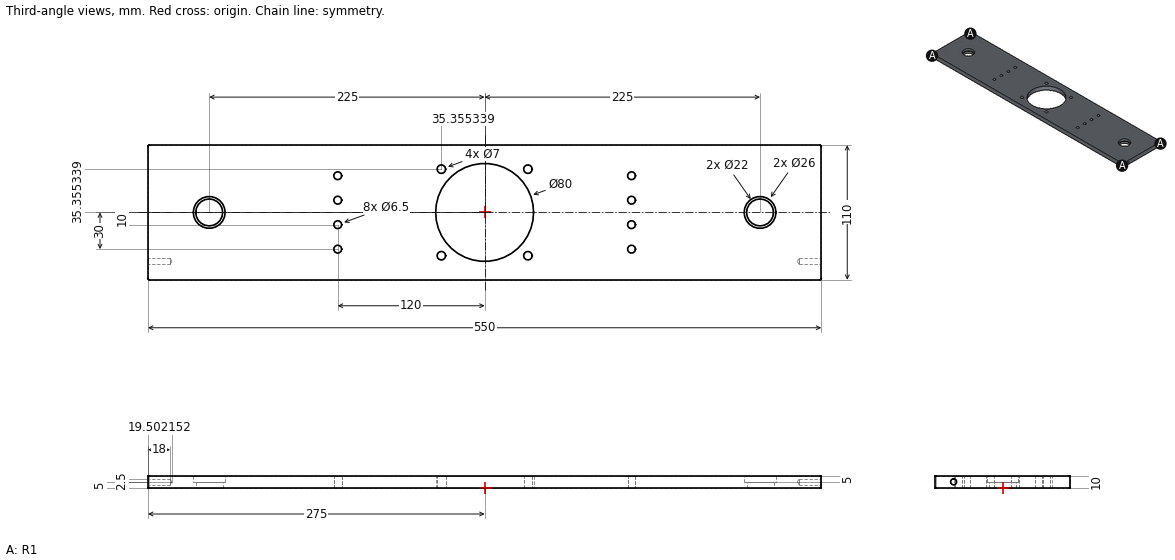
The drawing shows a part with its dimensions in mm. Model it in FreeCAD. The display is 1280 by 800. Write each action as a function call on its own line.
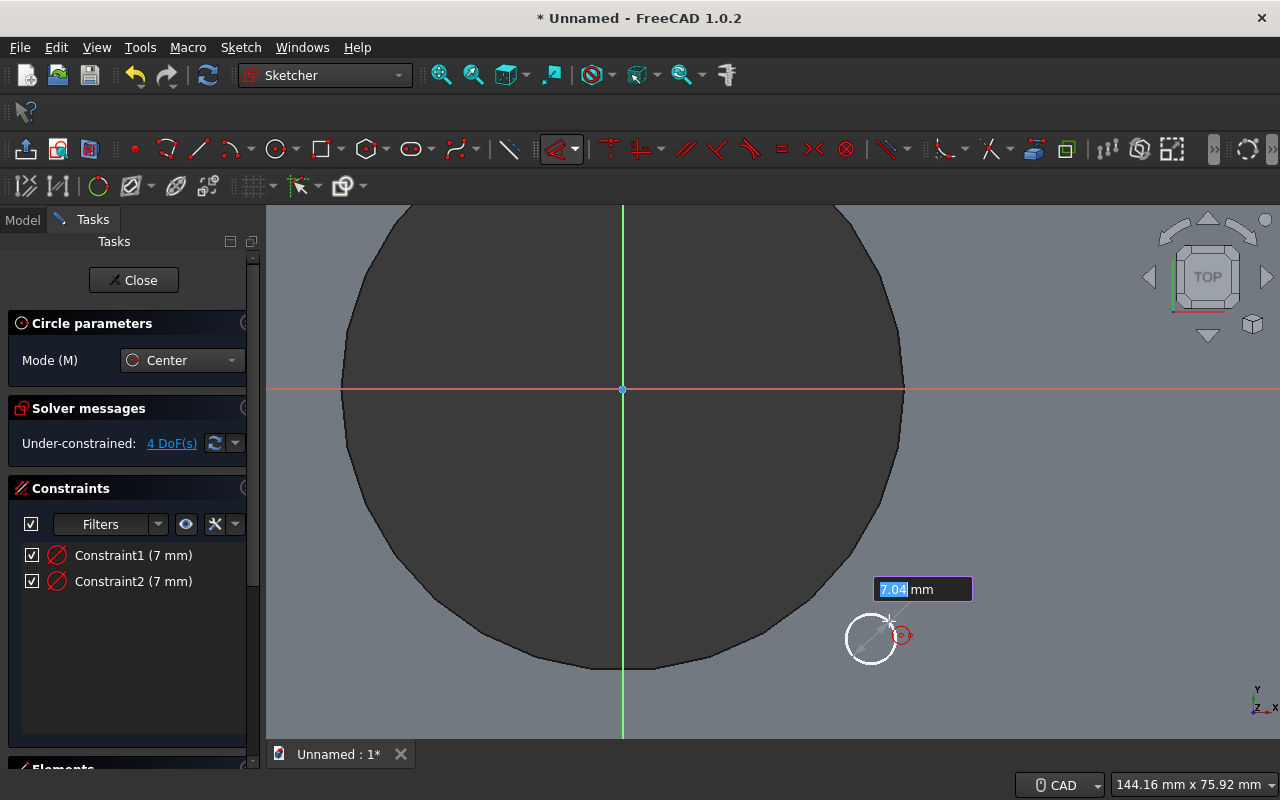
text(7)
key(Return)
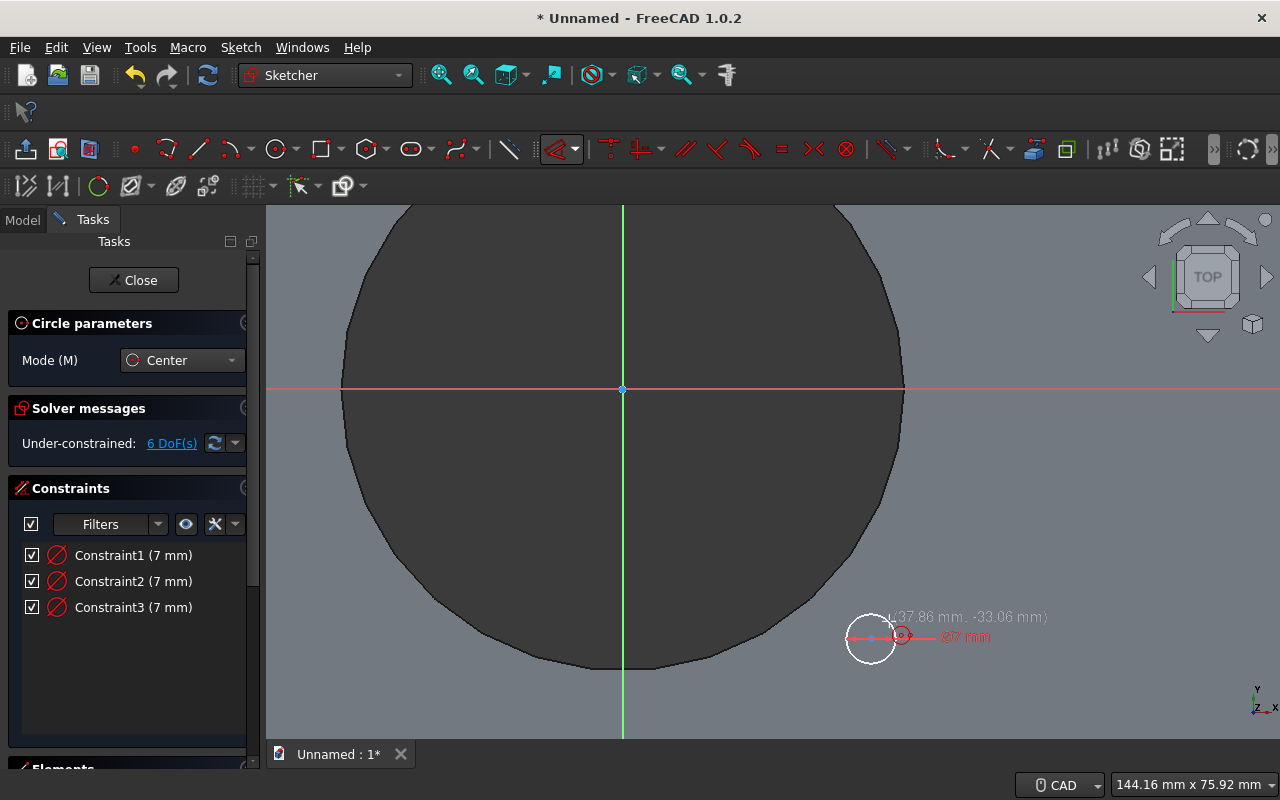
click(374, 638)
move(391, 621)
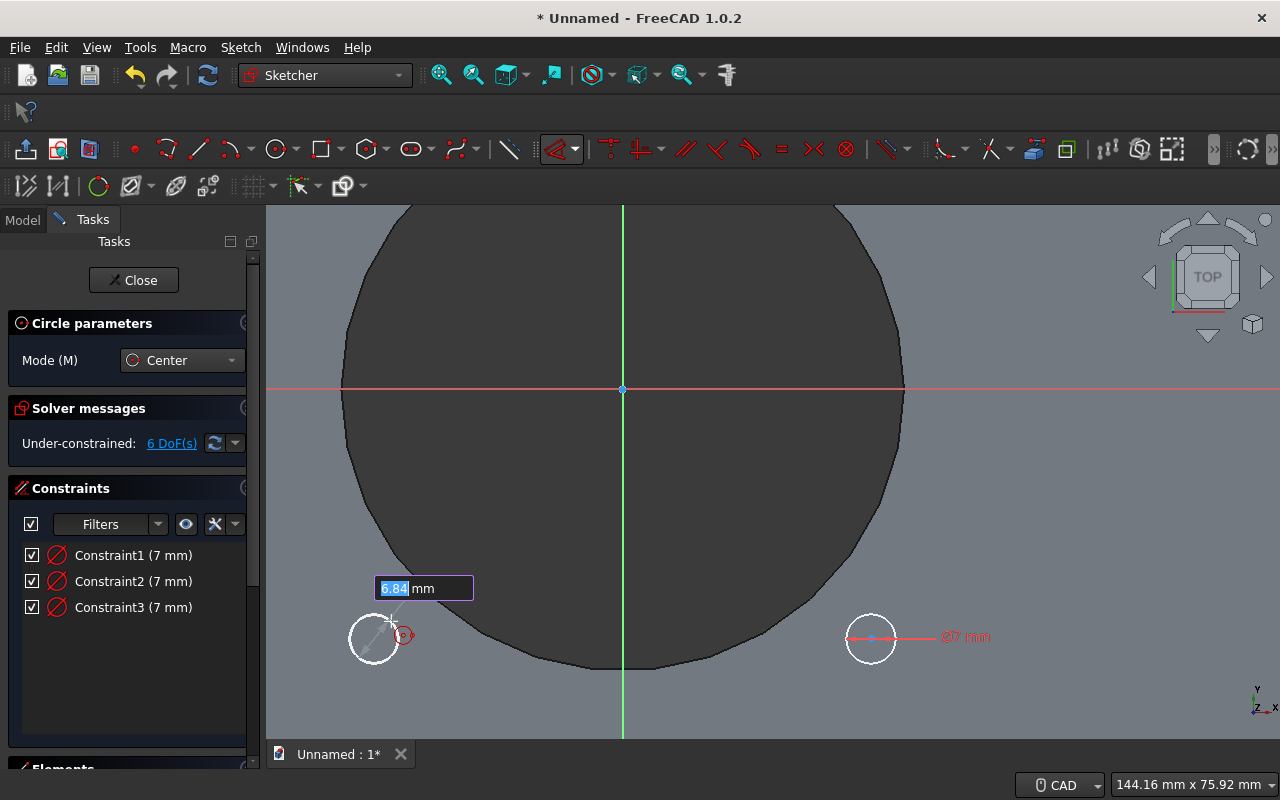
text(7)
key(Return)
key(Escape)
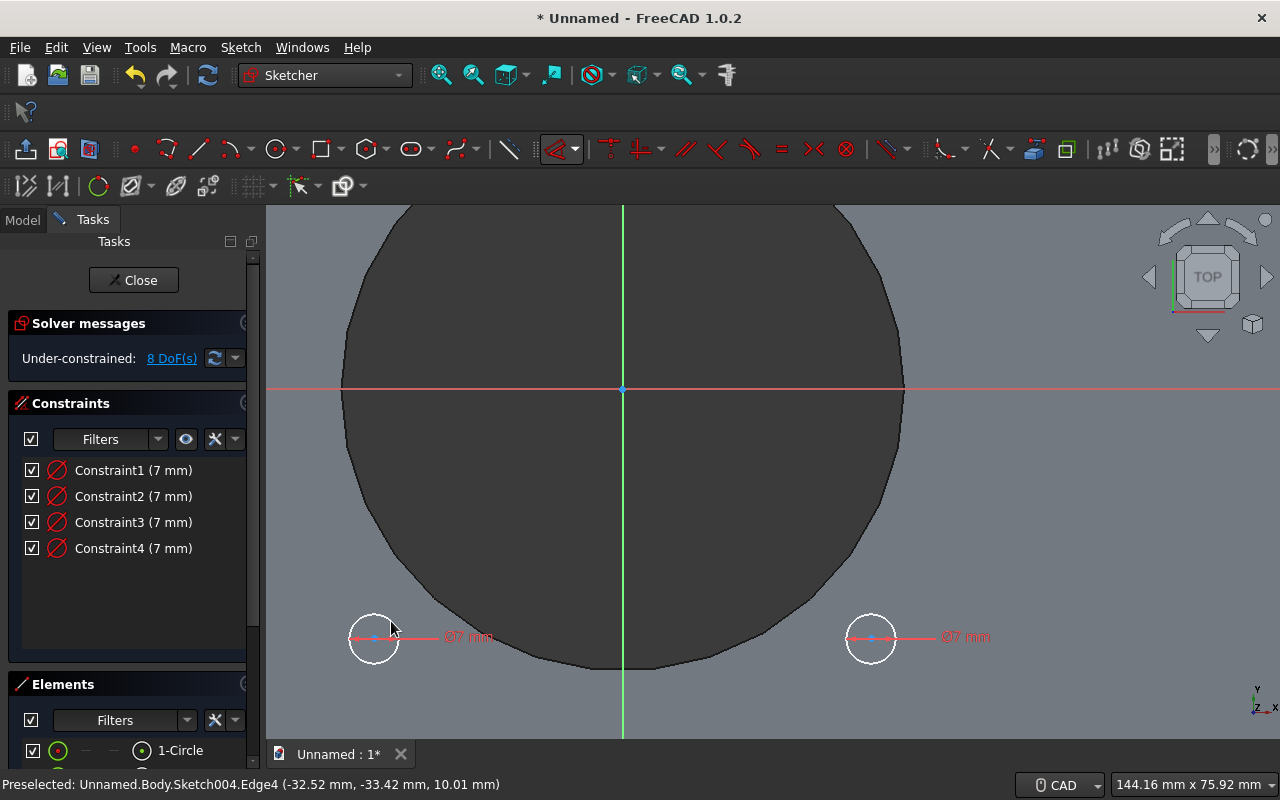
scroll(871, 640, down, 2)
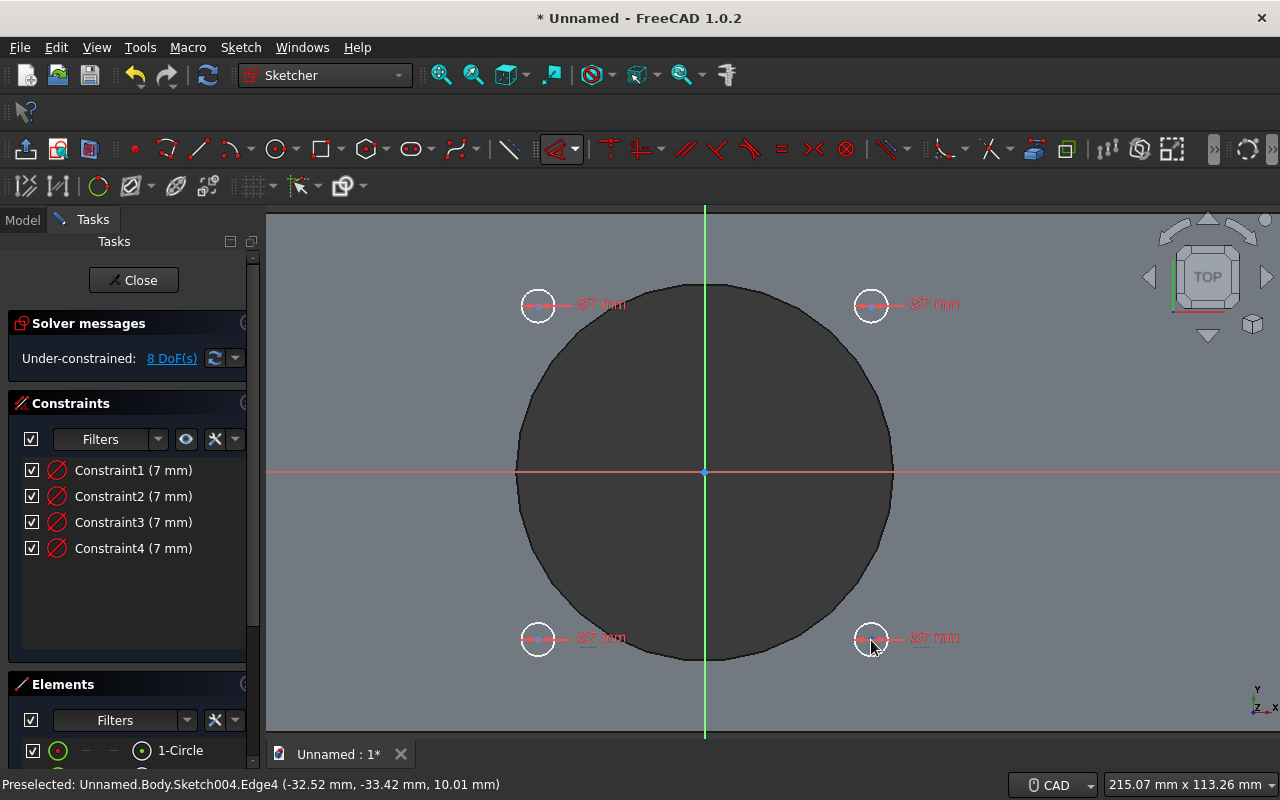
click(538, 306)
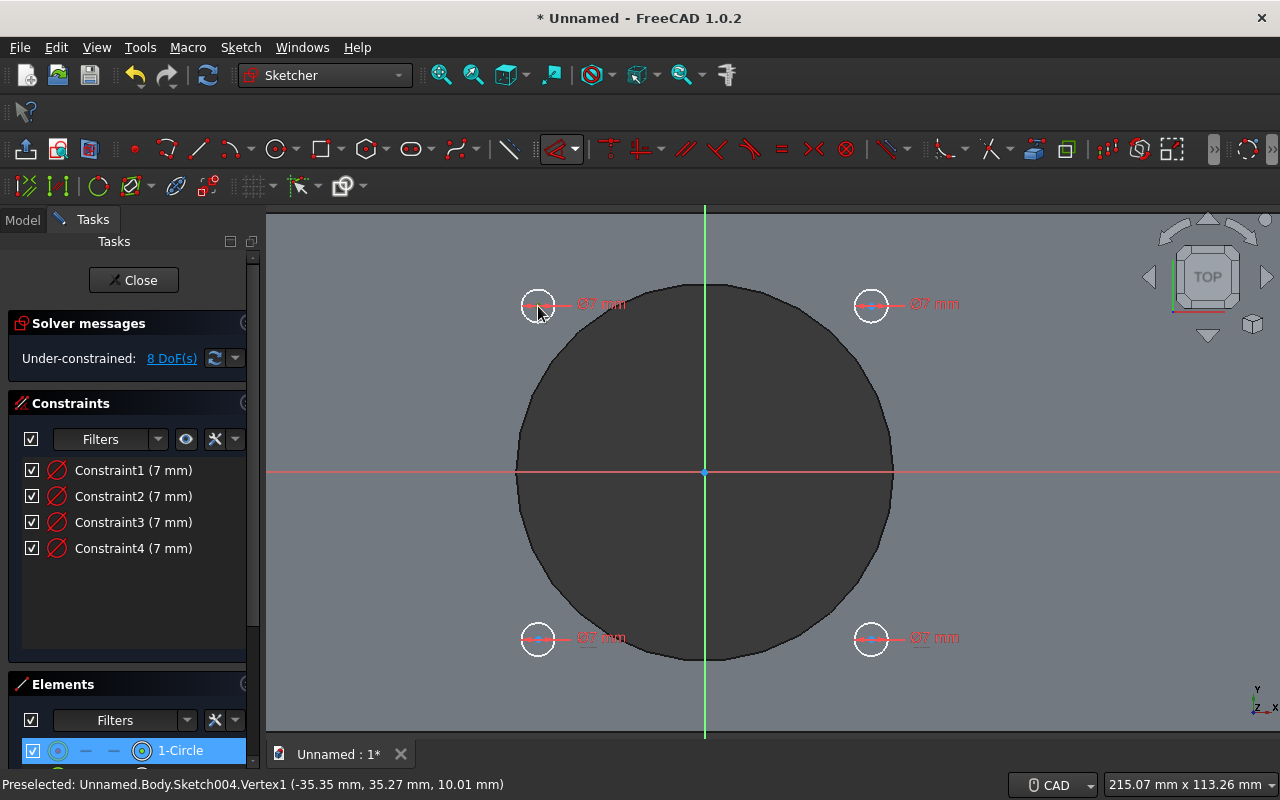
click(871, 306)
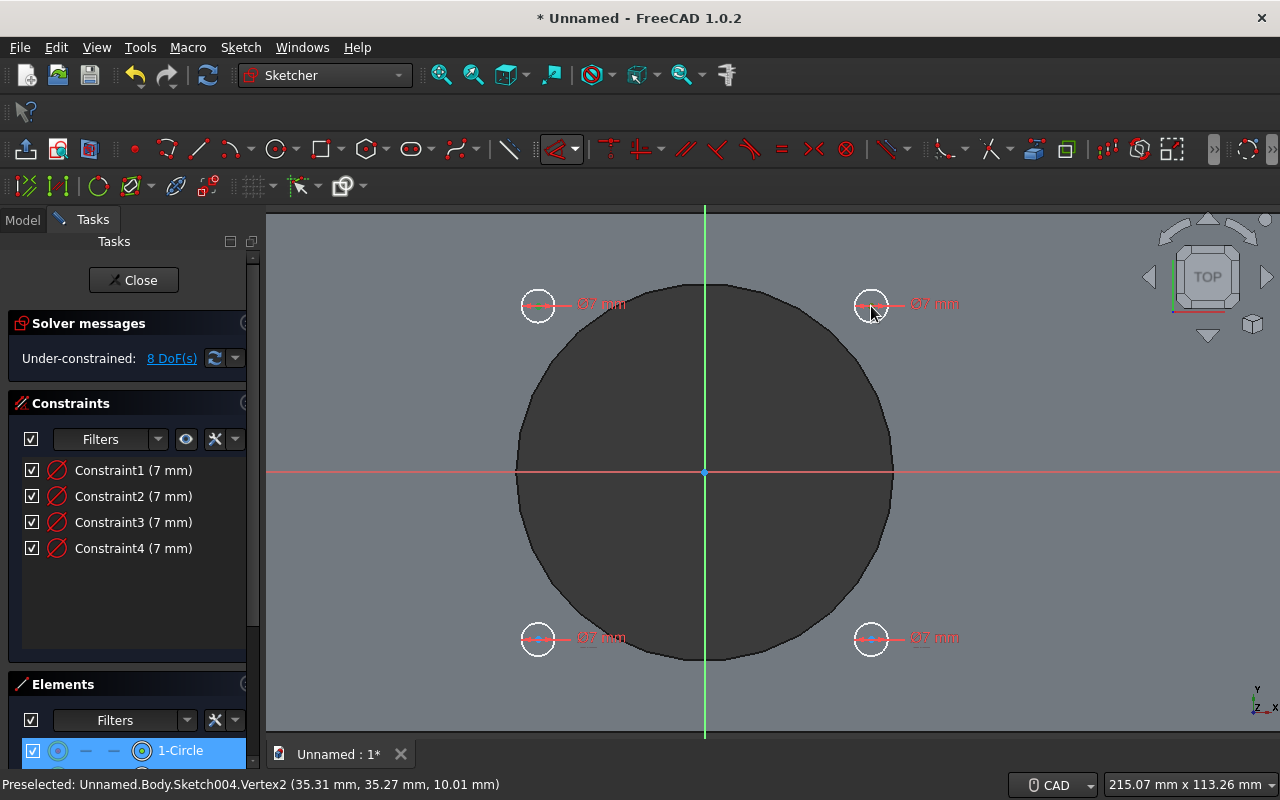
click(705, 677)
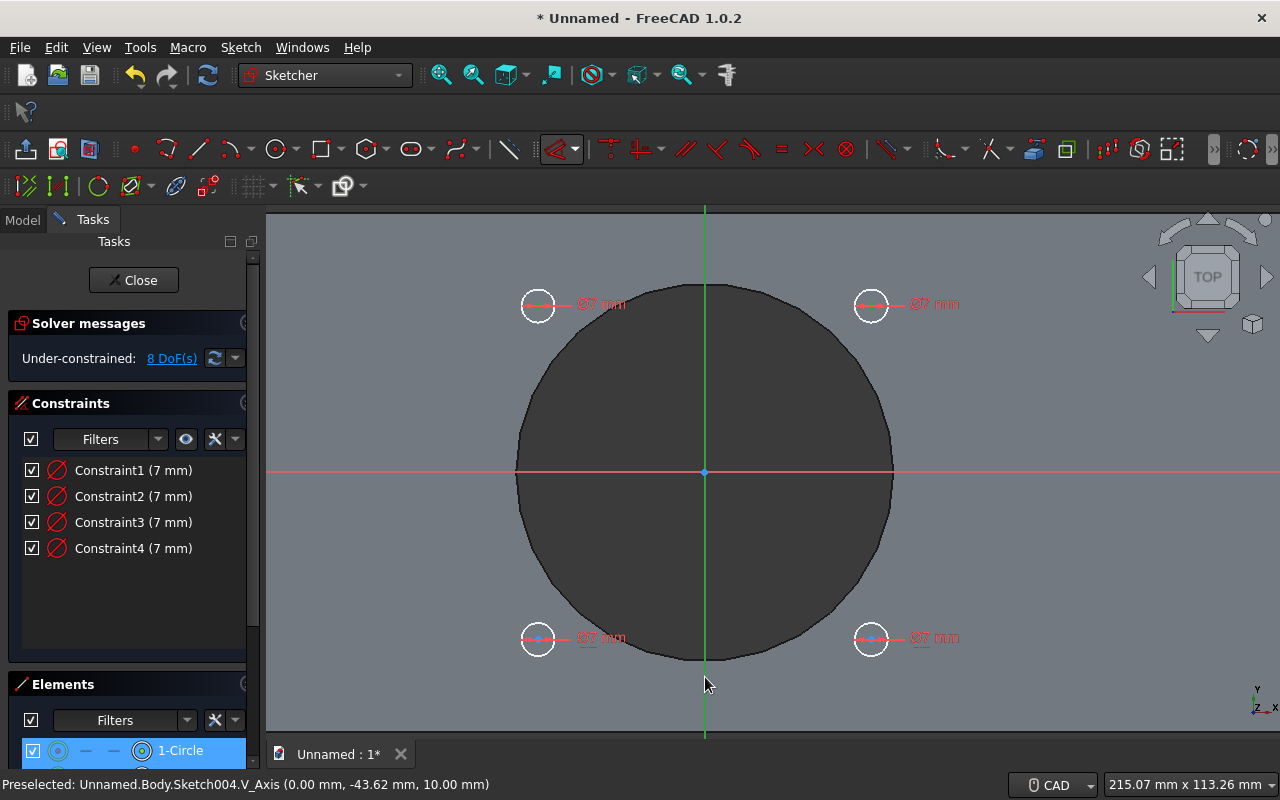
key(s)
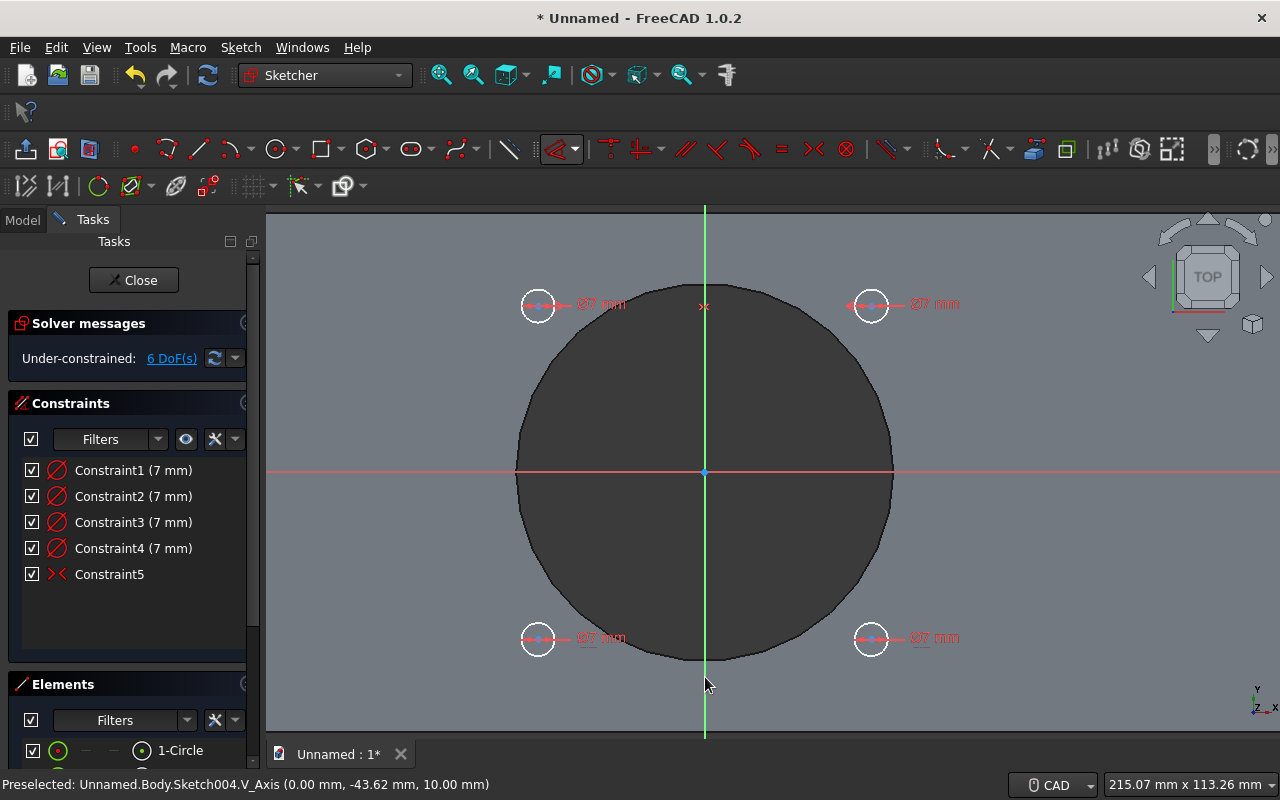
click(871, 306)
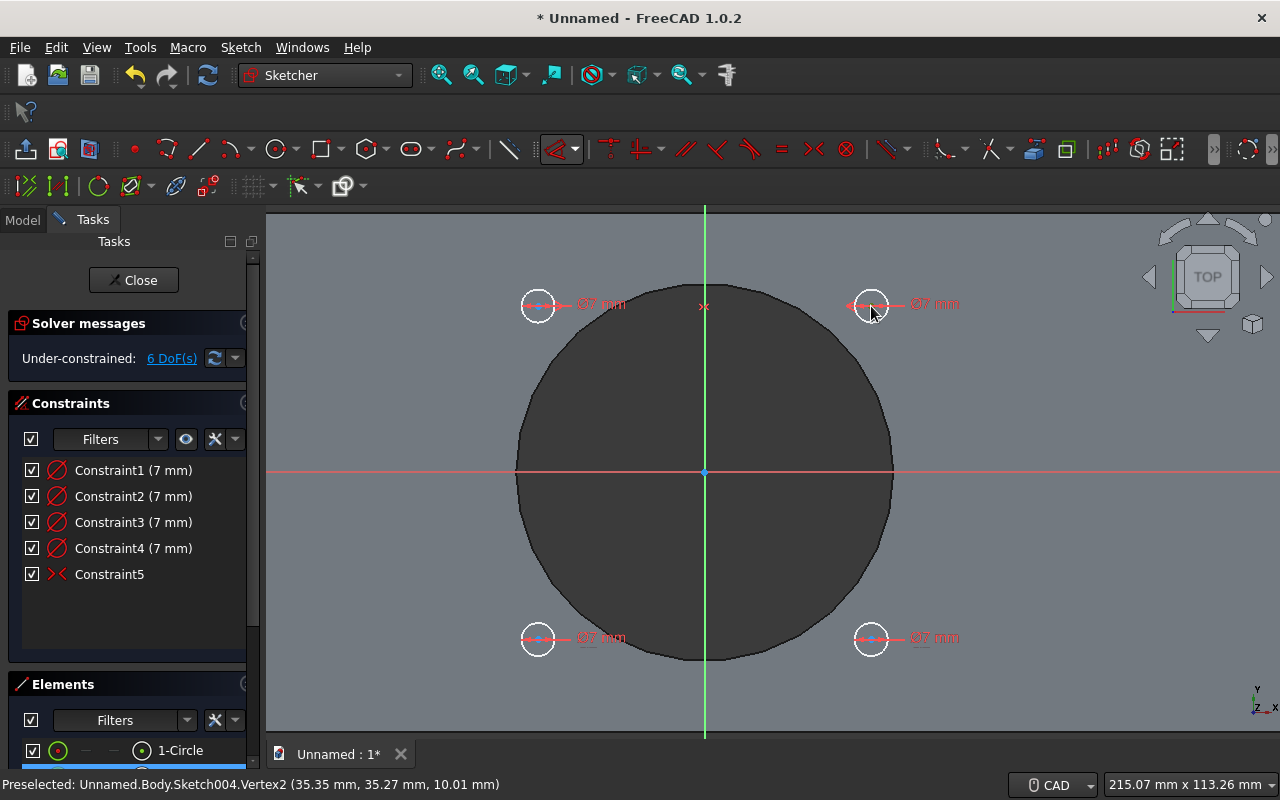
click(871, 640)